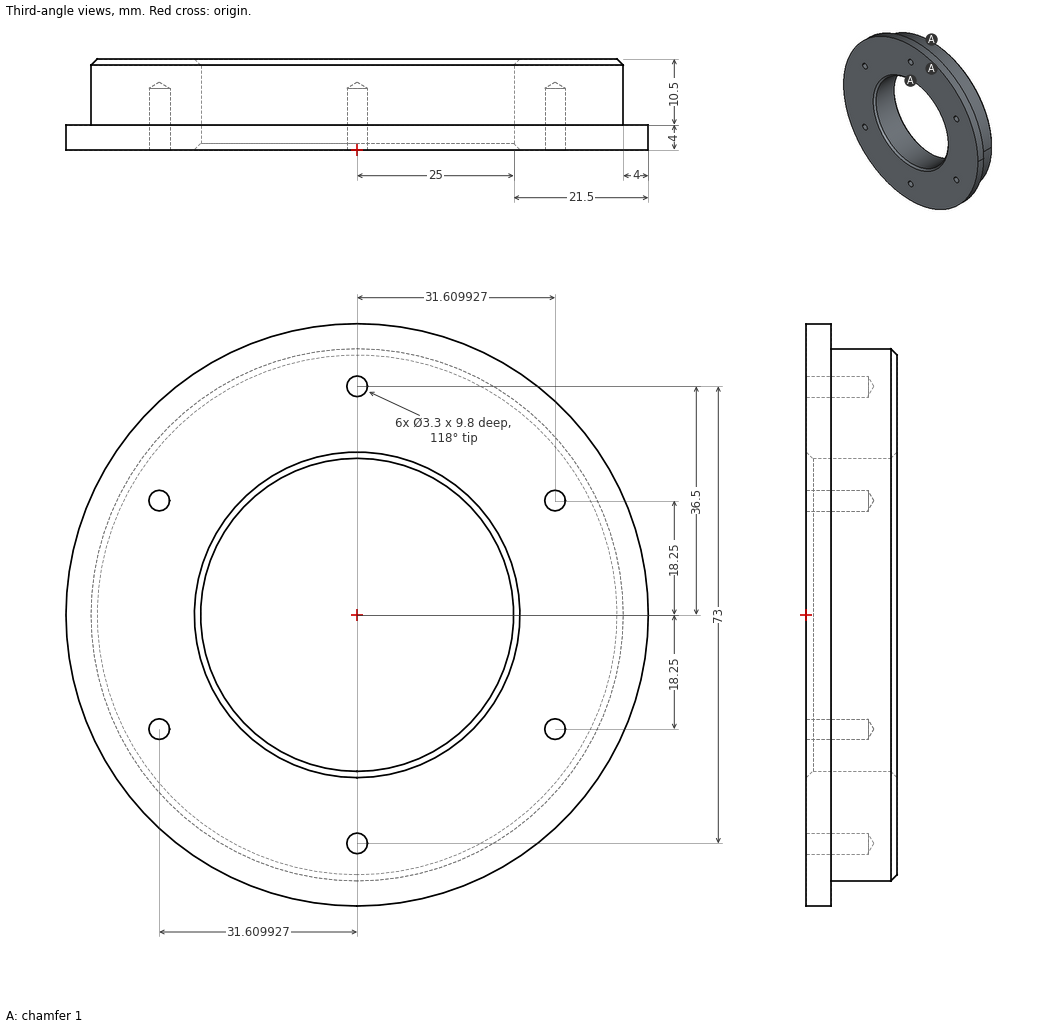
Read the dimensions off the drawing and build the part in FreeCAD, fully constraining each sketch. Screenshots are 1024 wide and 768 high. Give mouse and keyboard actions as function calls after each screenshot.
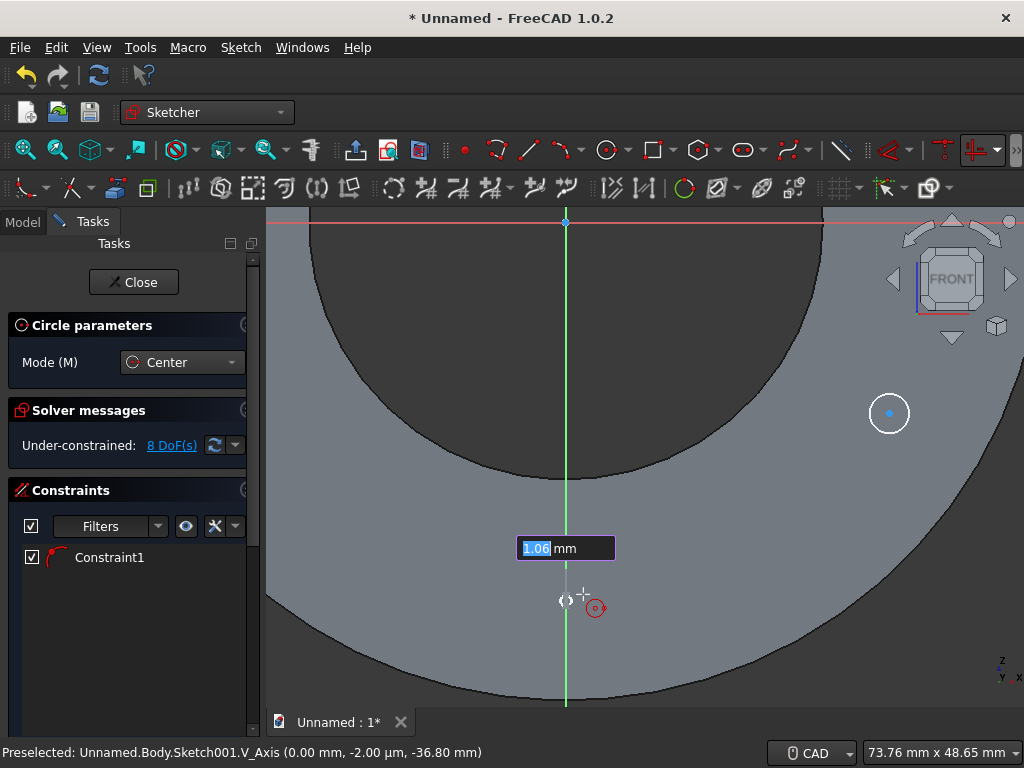
click(582, 592)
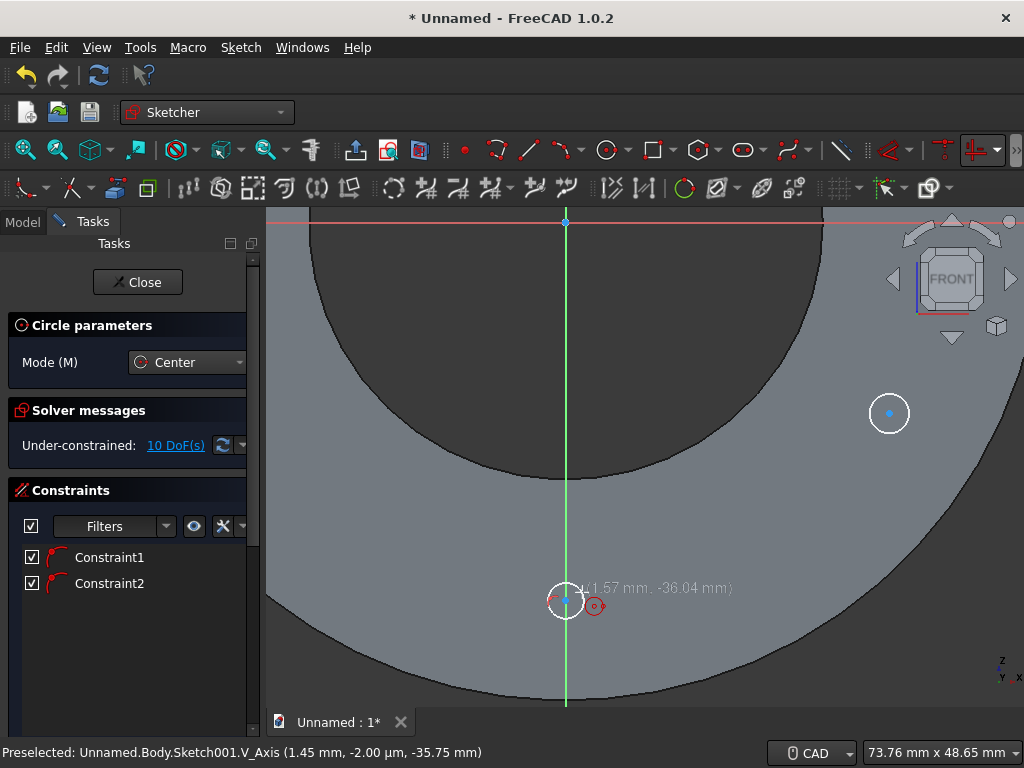
scroll(583, 593, down, 5)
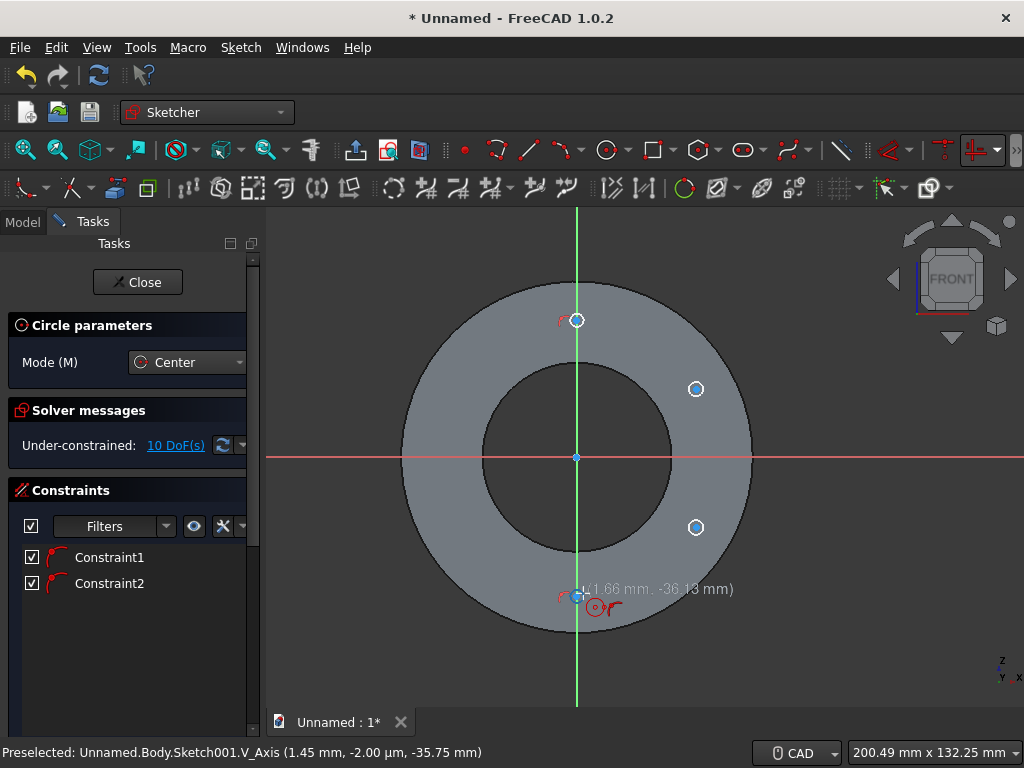
scroll(457, 526, up, 7)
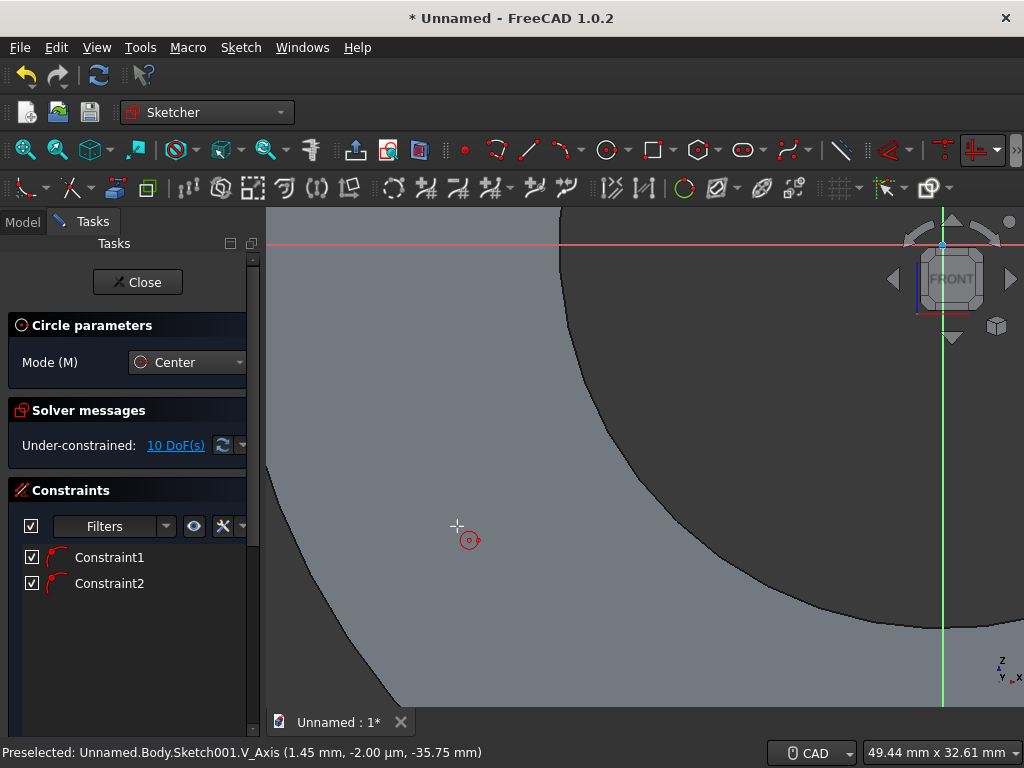
scroll(457, 526, down, 7)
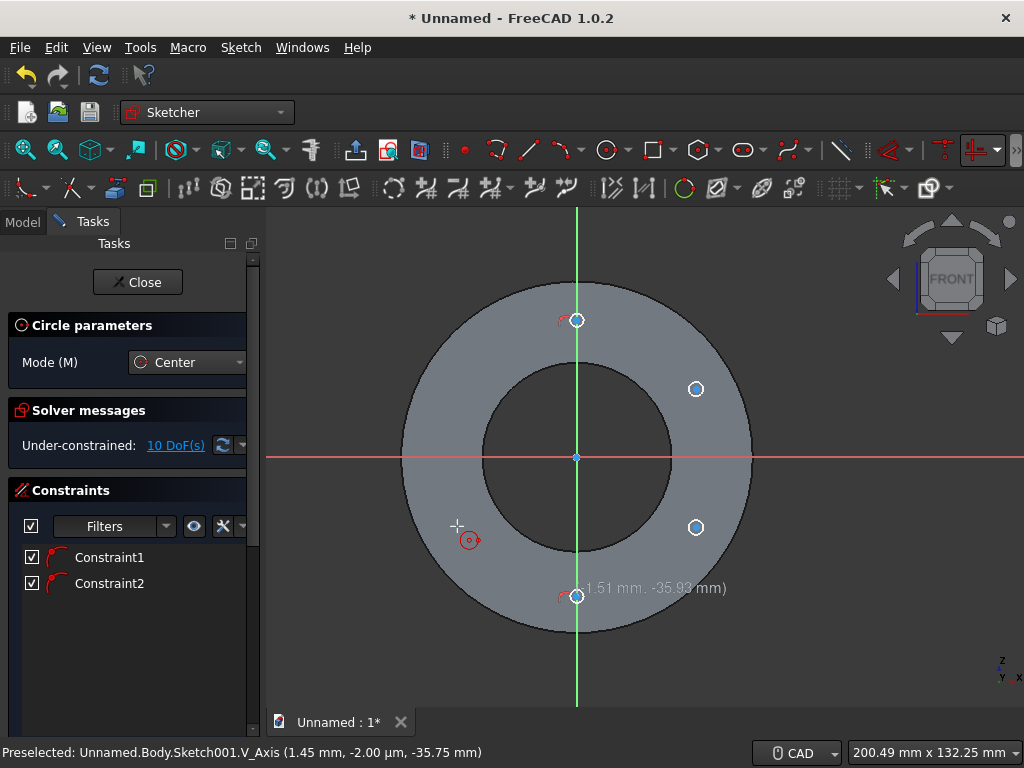
click(457, 526)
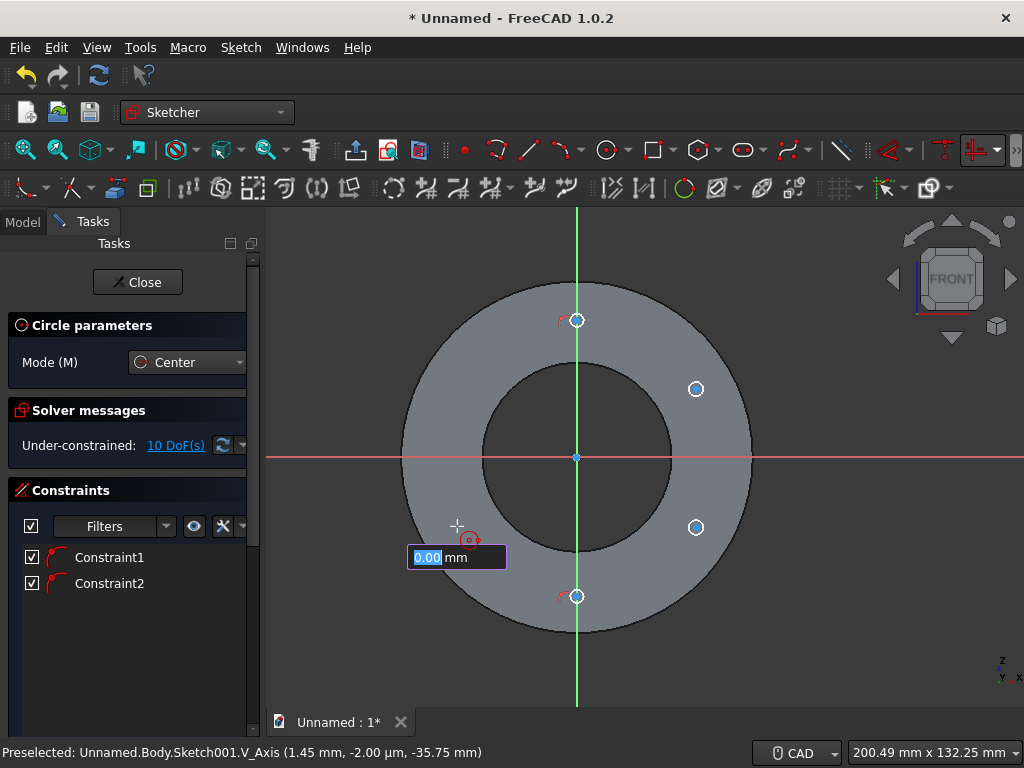
scroll(462, 522, up, 5)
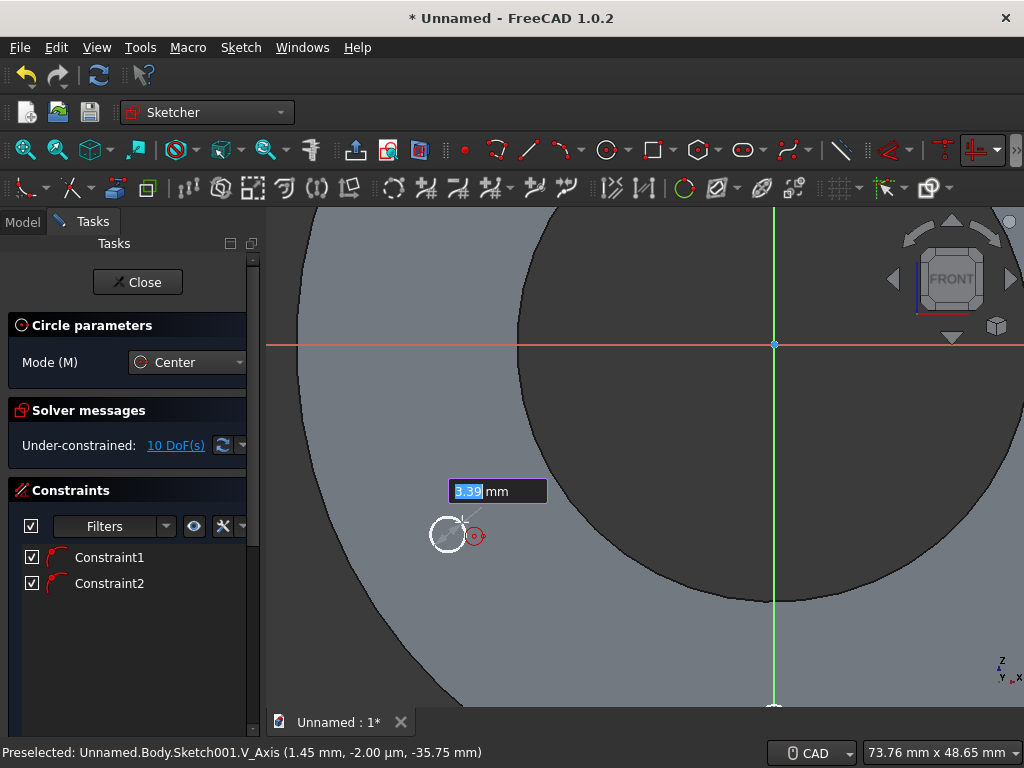
click(461, 520)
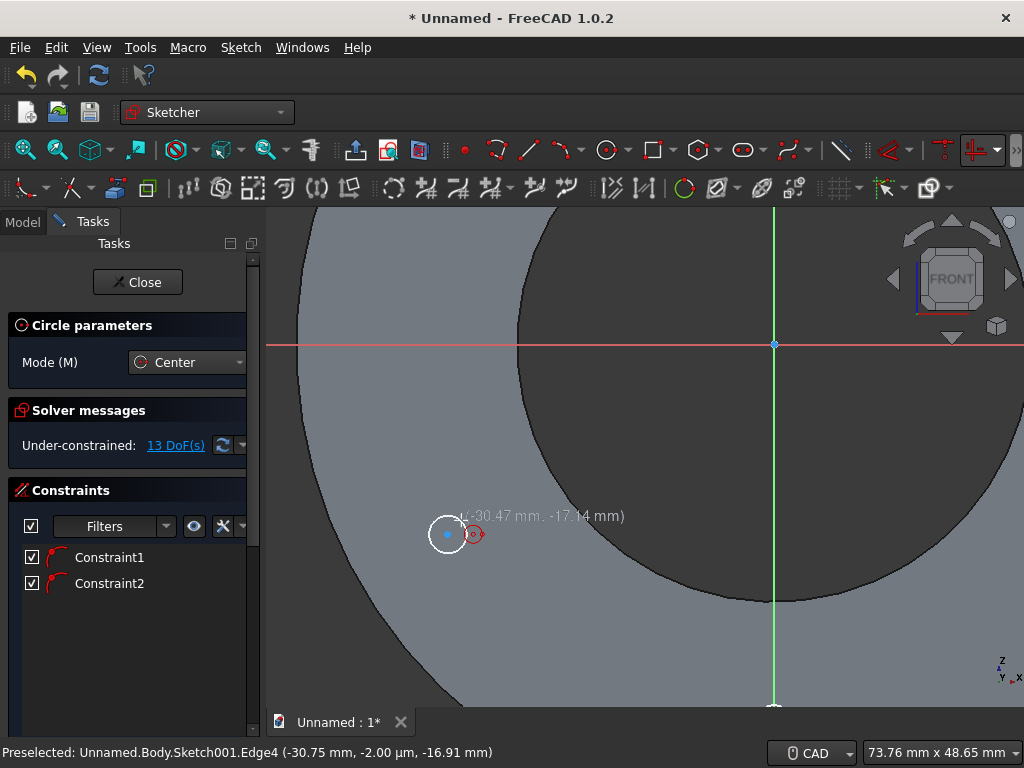
scroll(462, 522, down, 5)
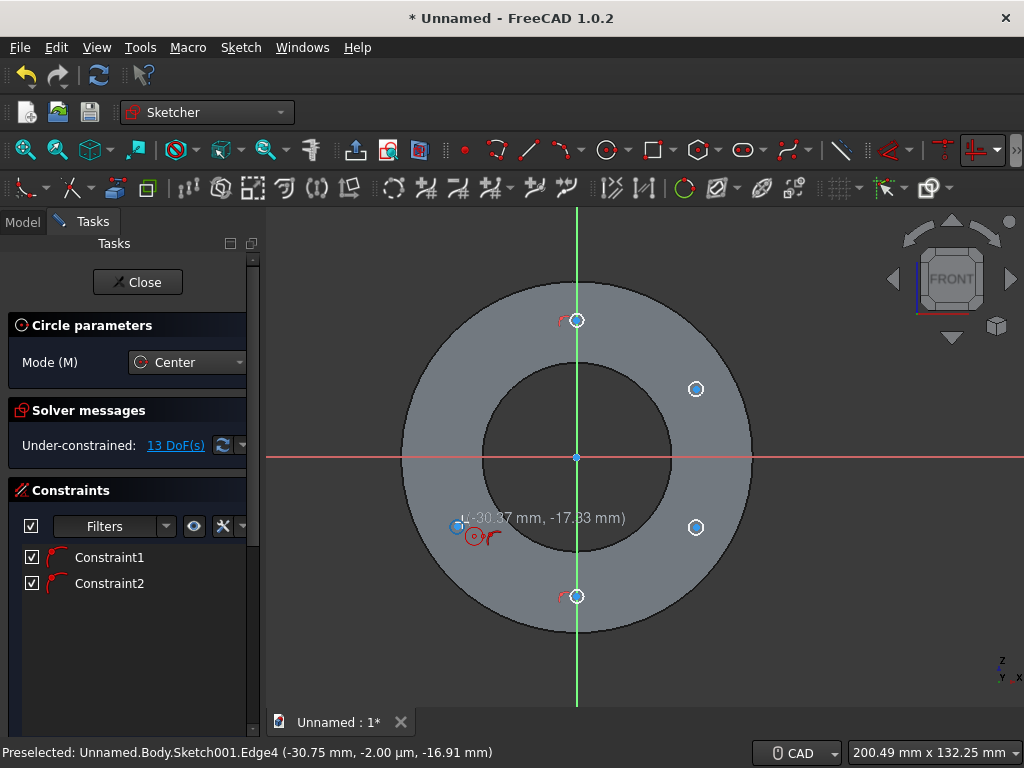
scroll(457, 388, up, 7)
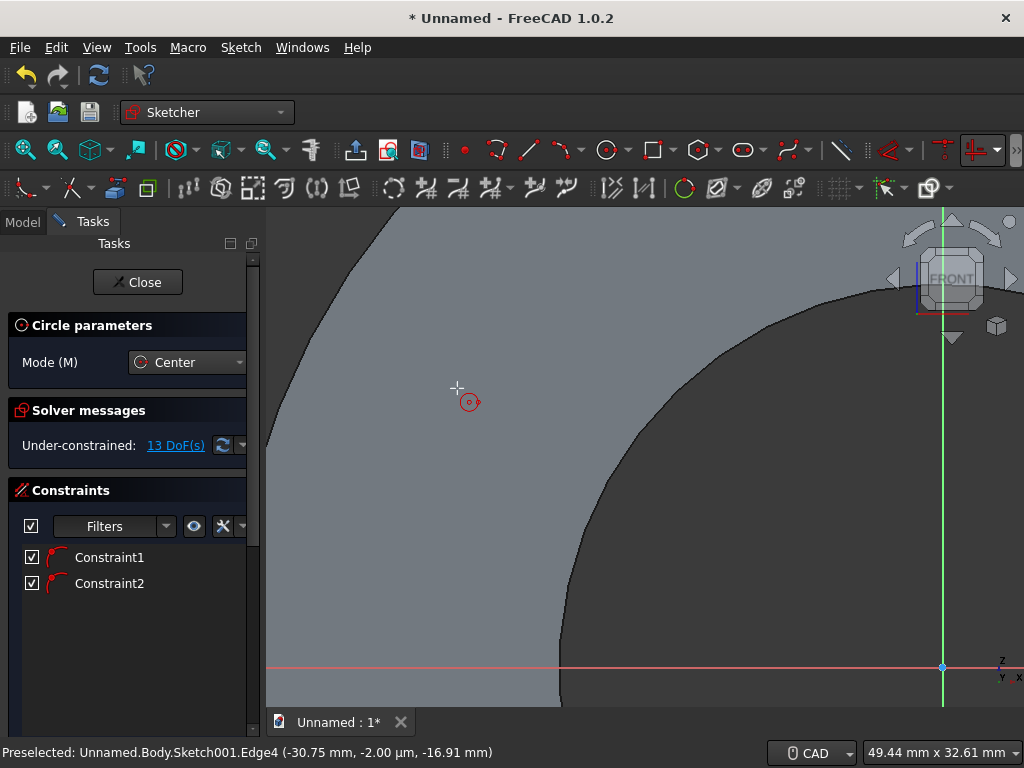
scroll(457, 388, down, 7)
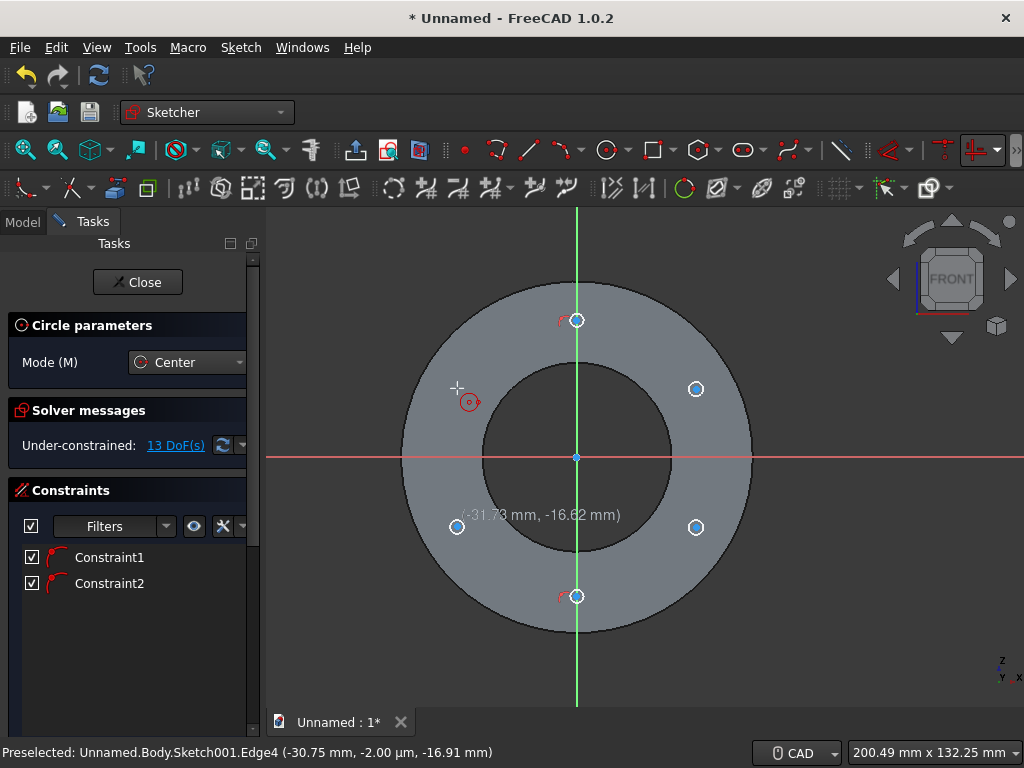
click(457, 388)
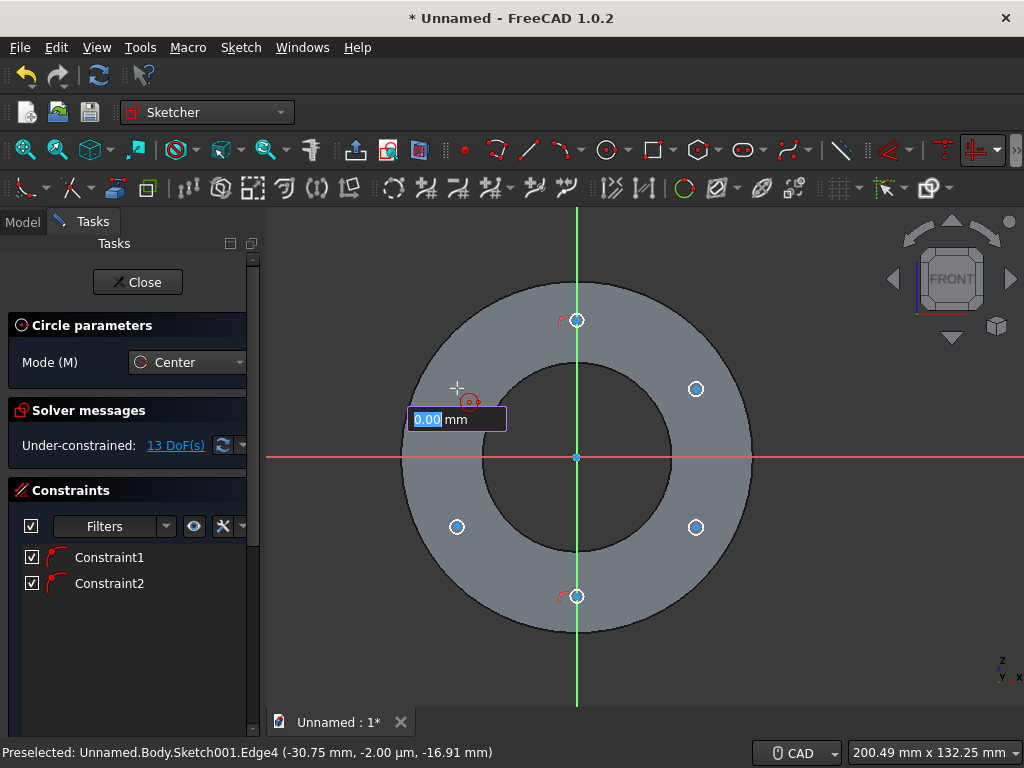
scroll(462, 384, up, 5)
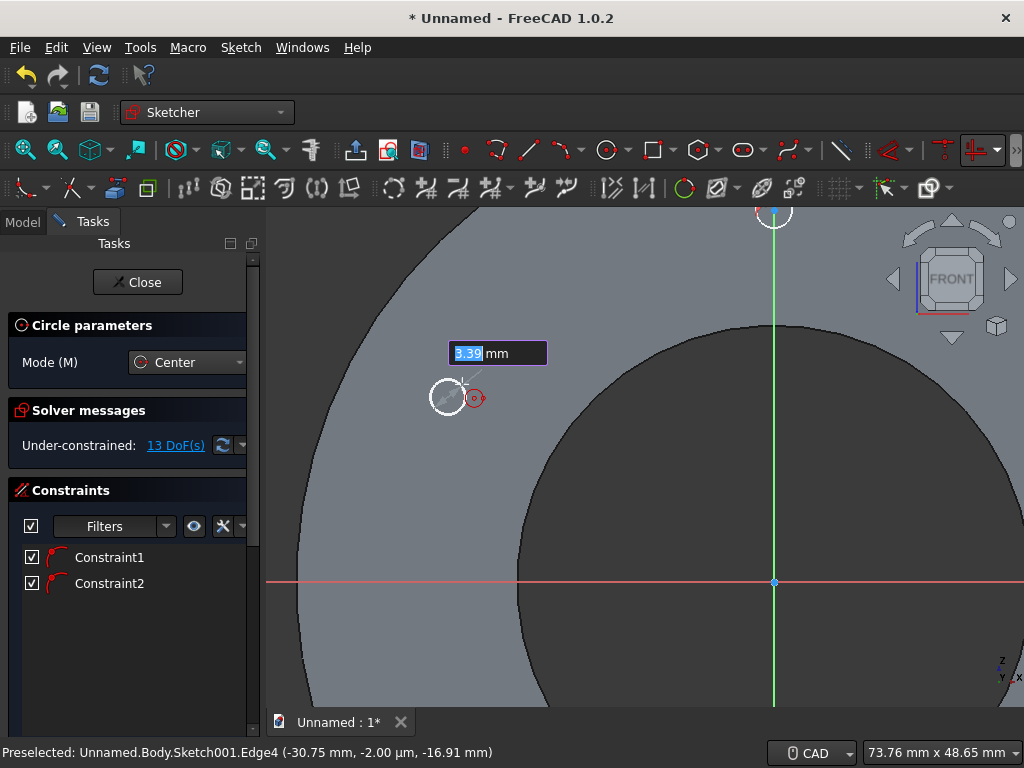
click(461, 383)
key(Escape)